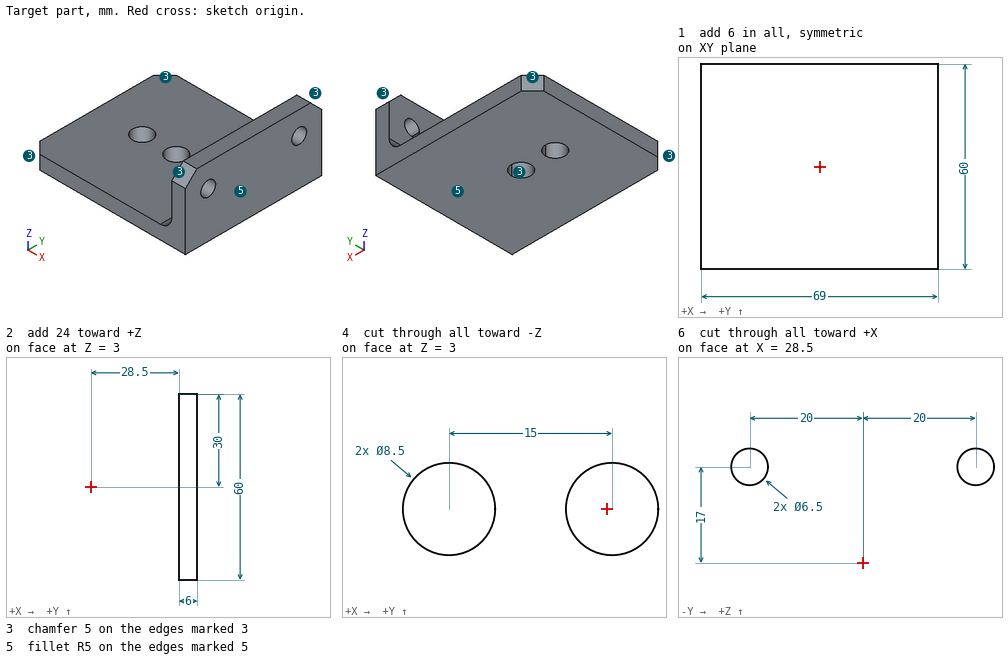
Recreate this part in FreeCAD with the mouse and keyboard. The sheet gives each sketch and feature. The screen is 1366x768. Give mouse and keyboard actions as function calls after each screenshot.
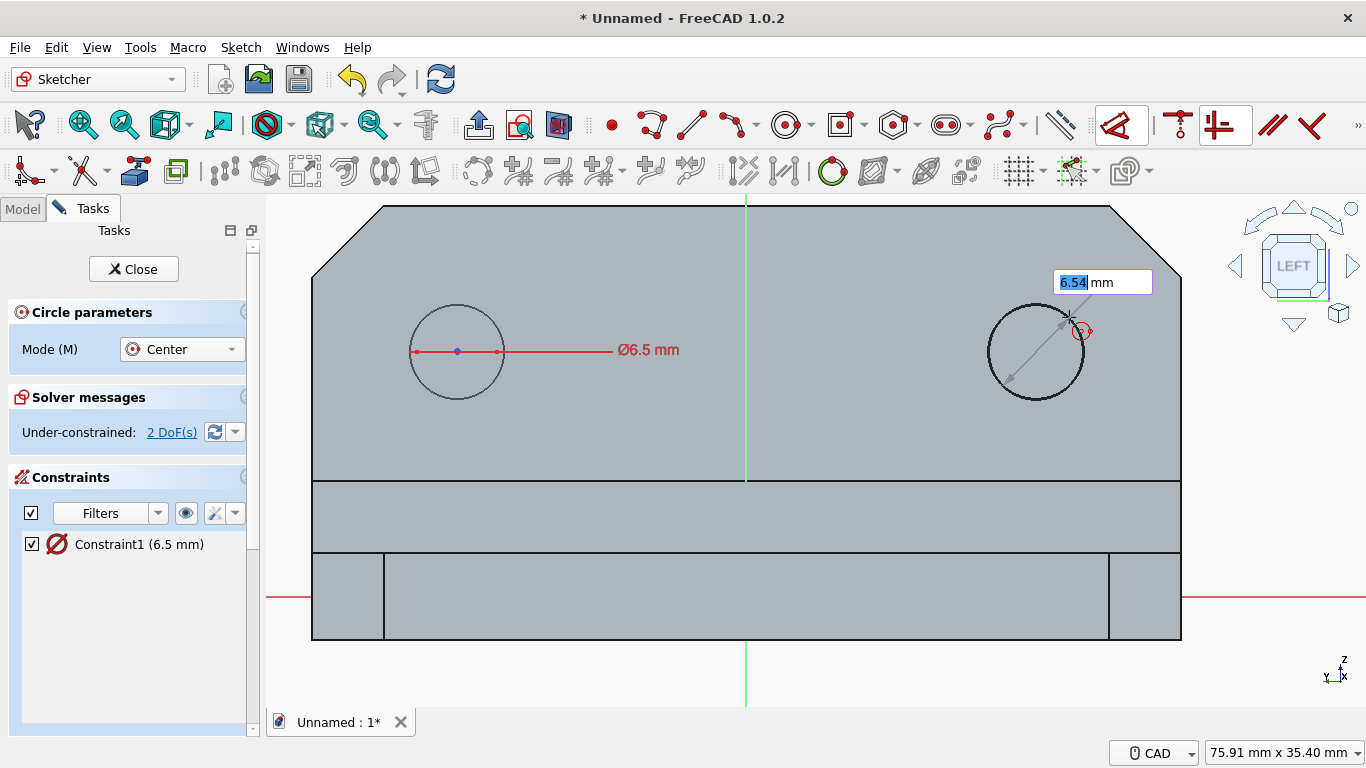
text(6.5)
key(Return)
key(Escape)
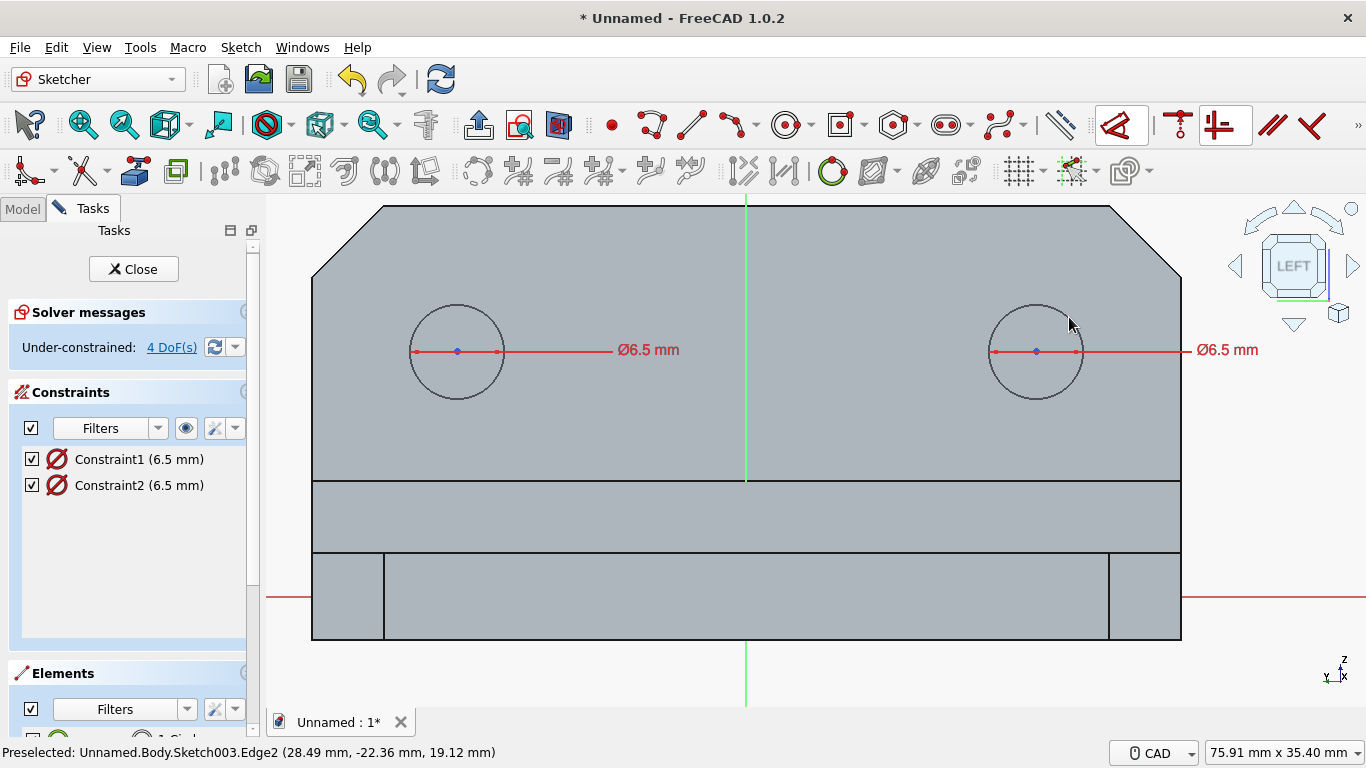
click(457, 352)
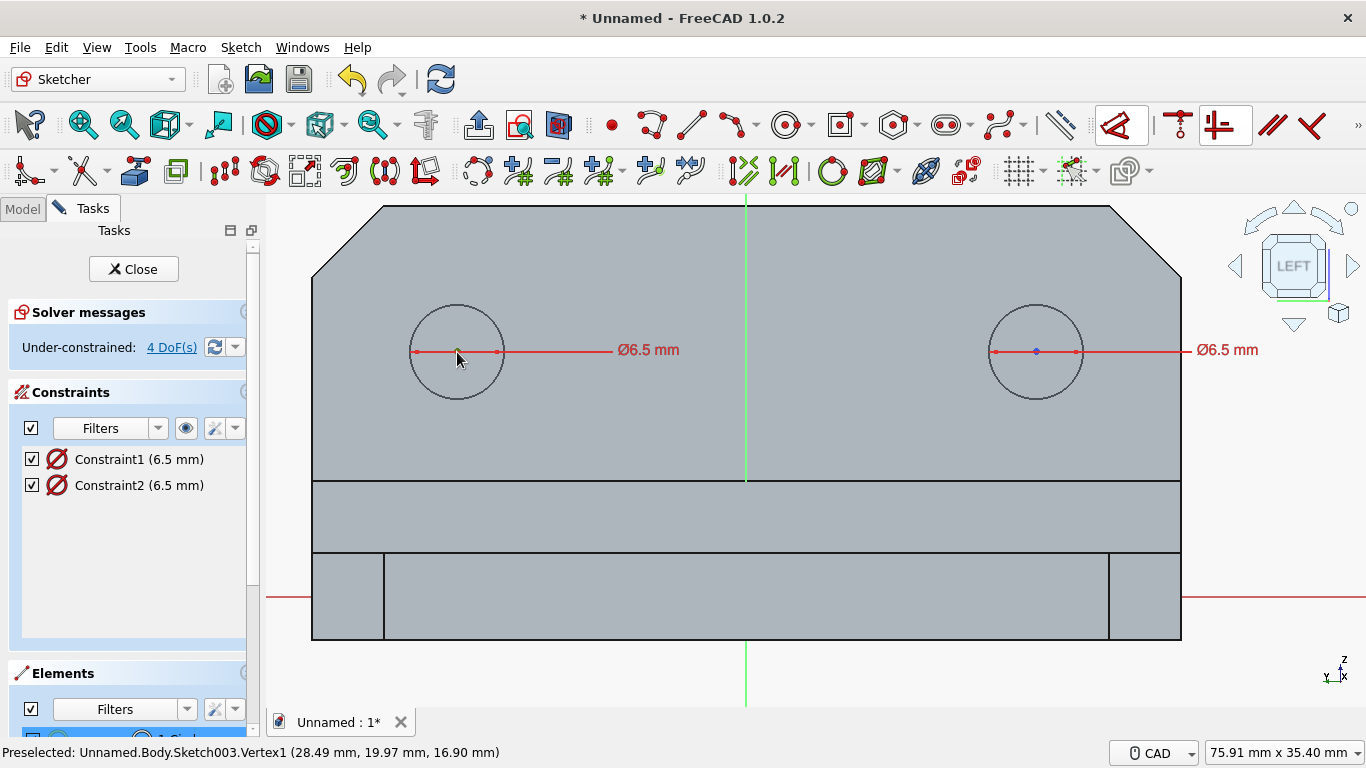
click(1036, 352)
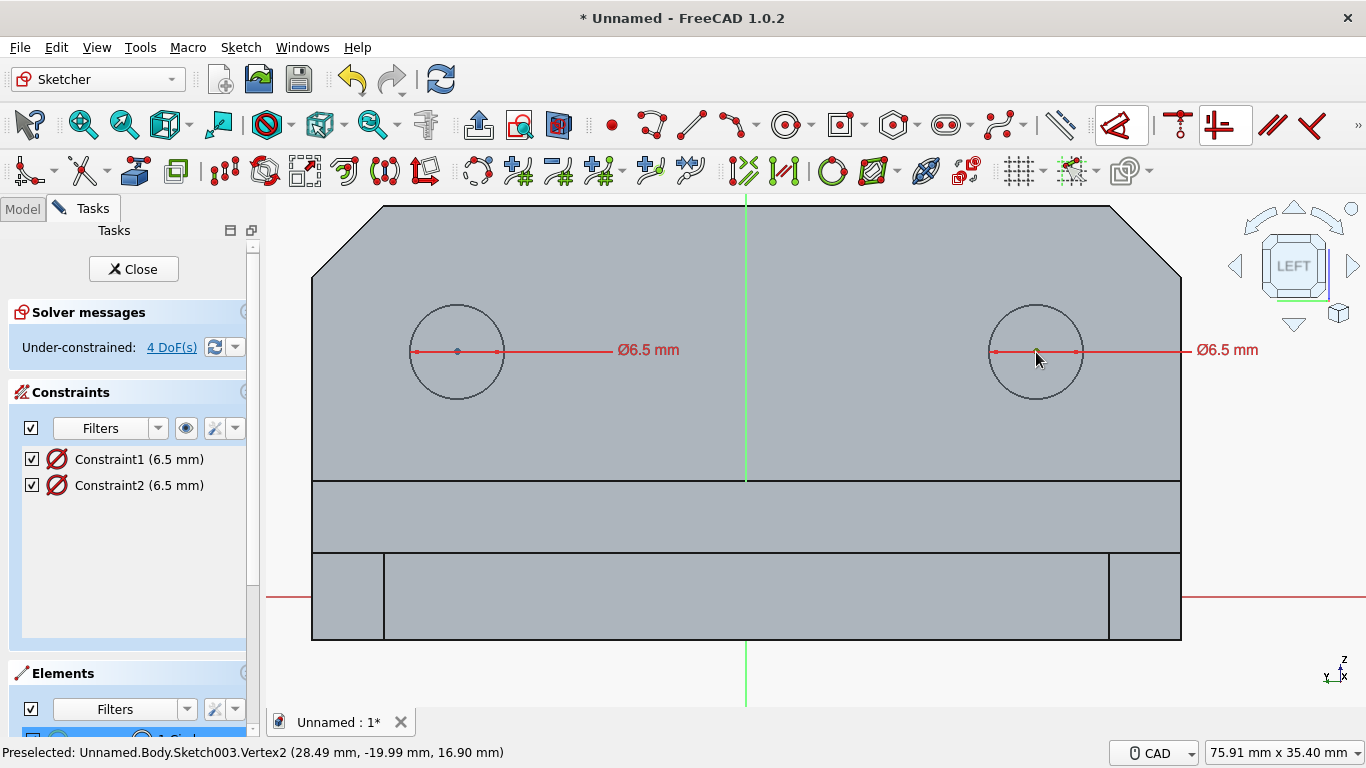
key(h)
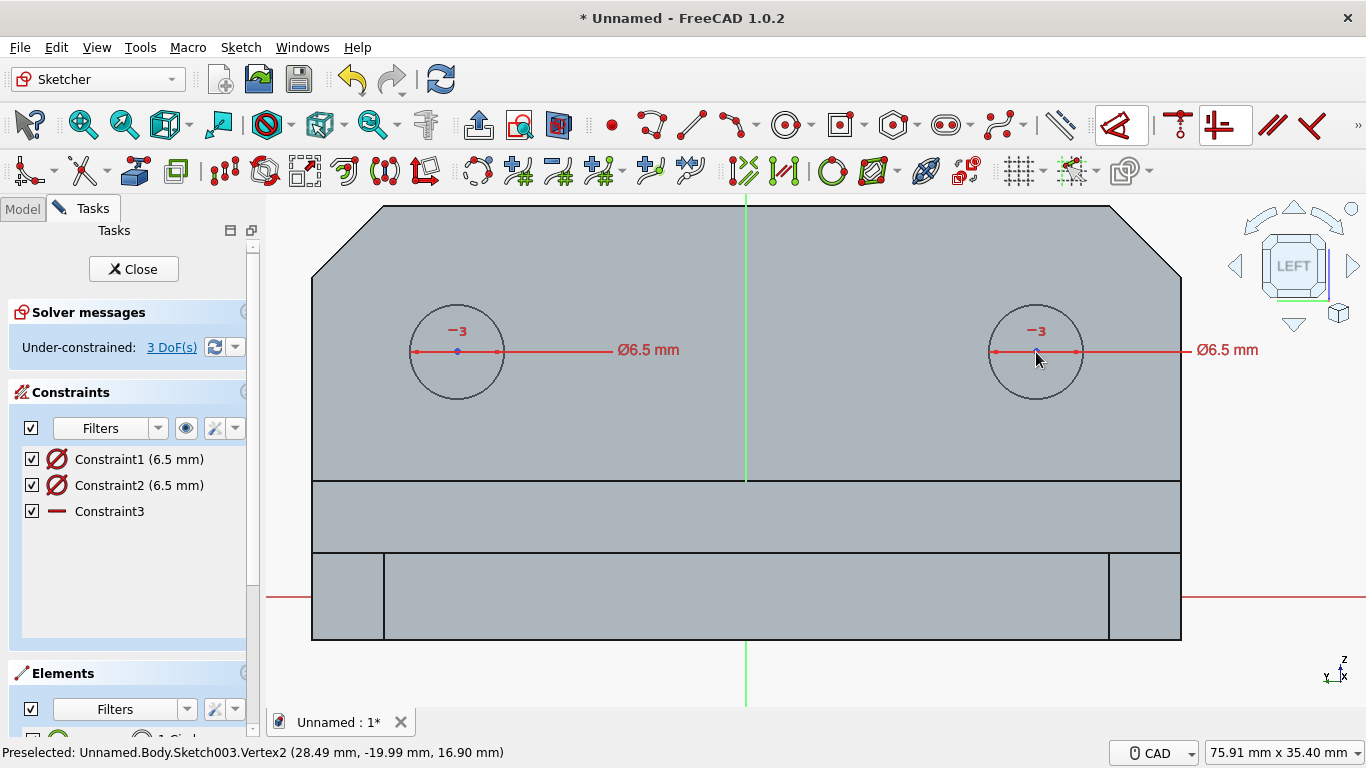
click(457, 352)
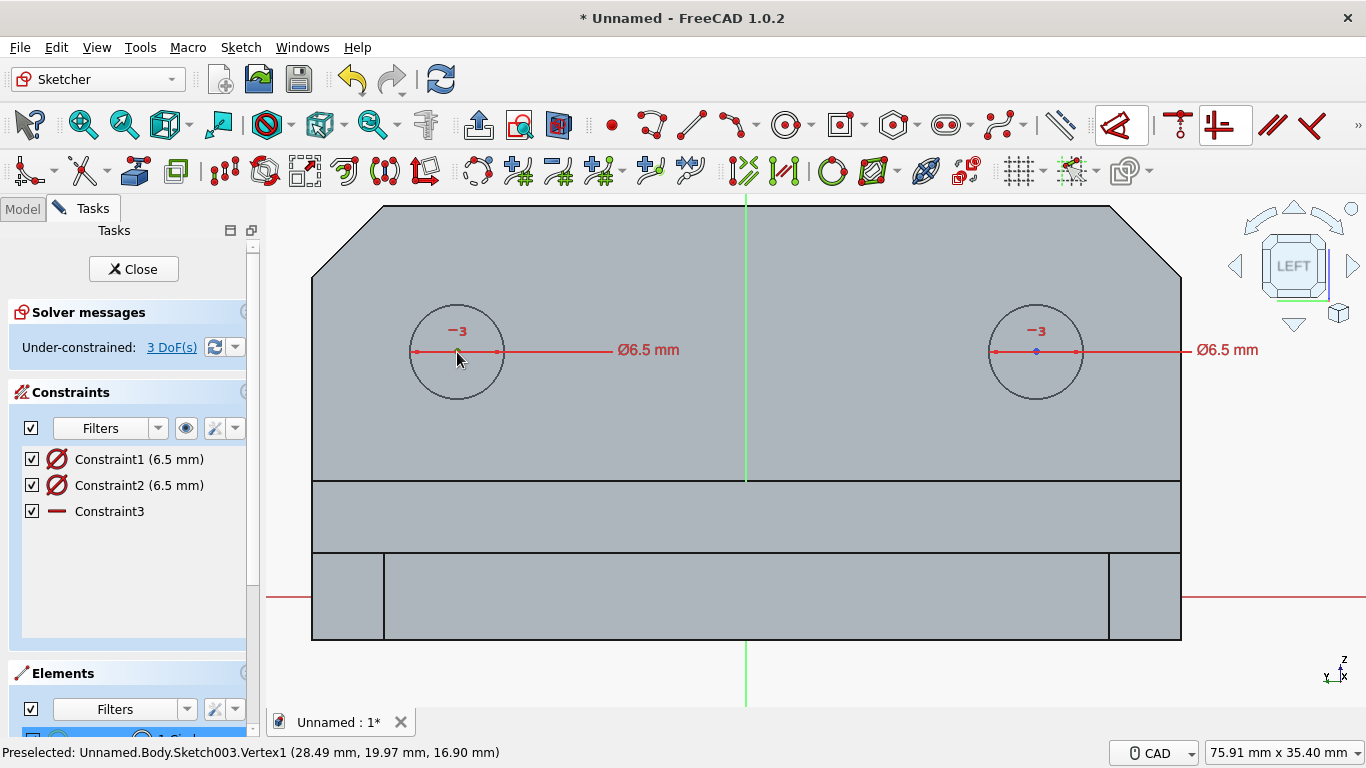
click(1142, 126)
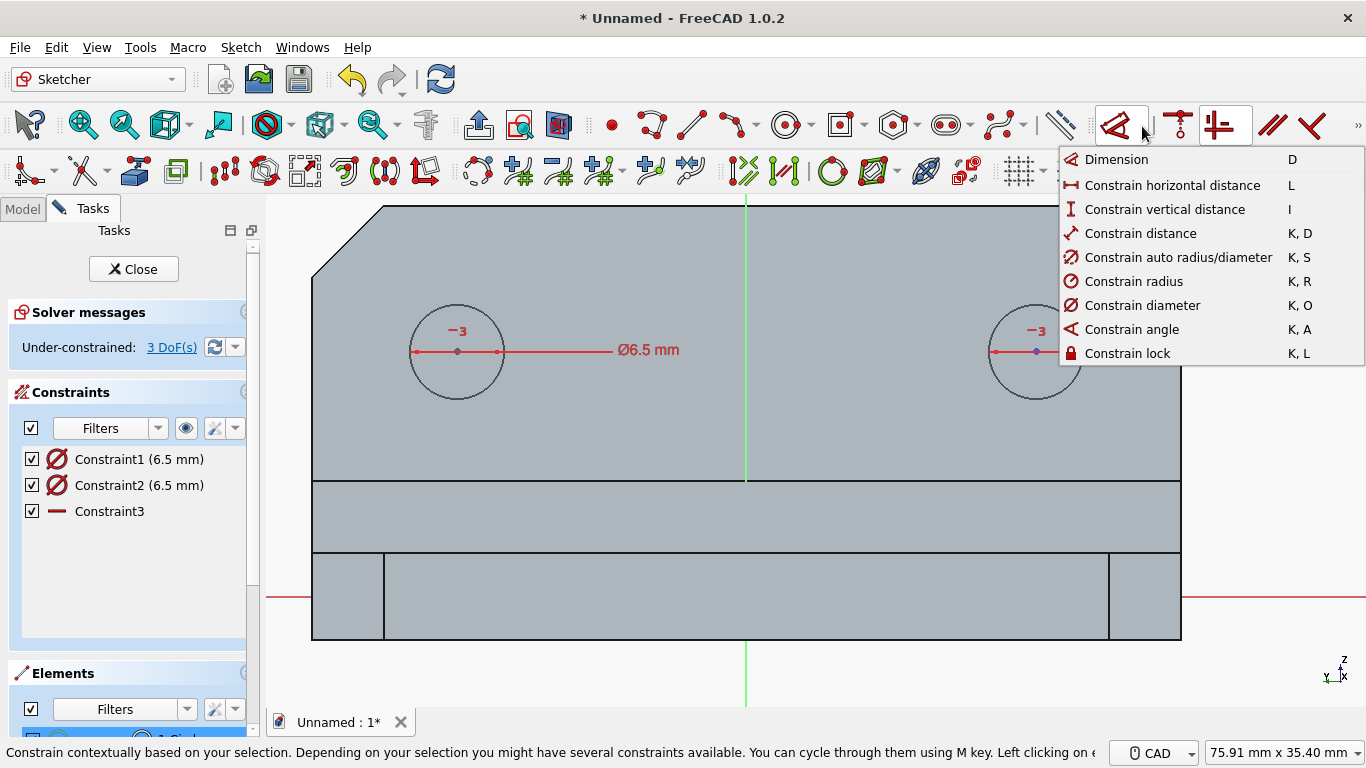
click(1212, 185)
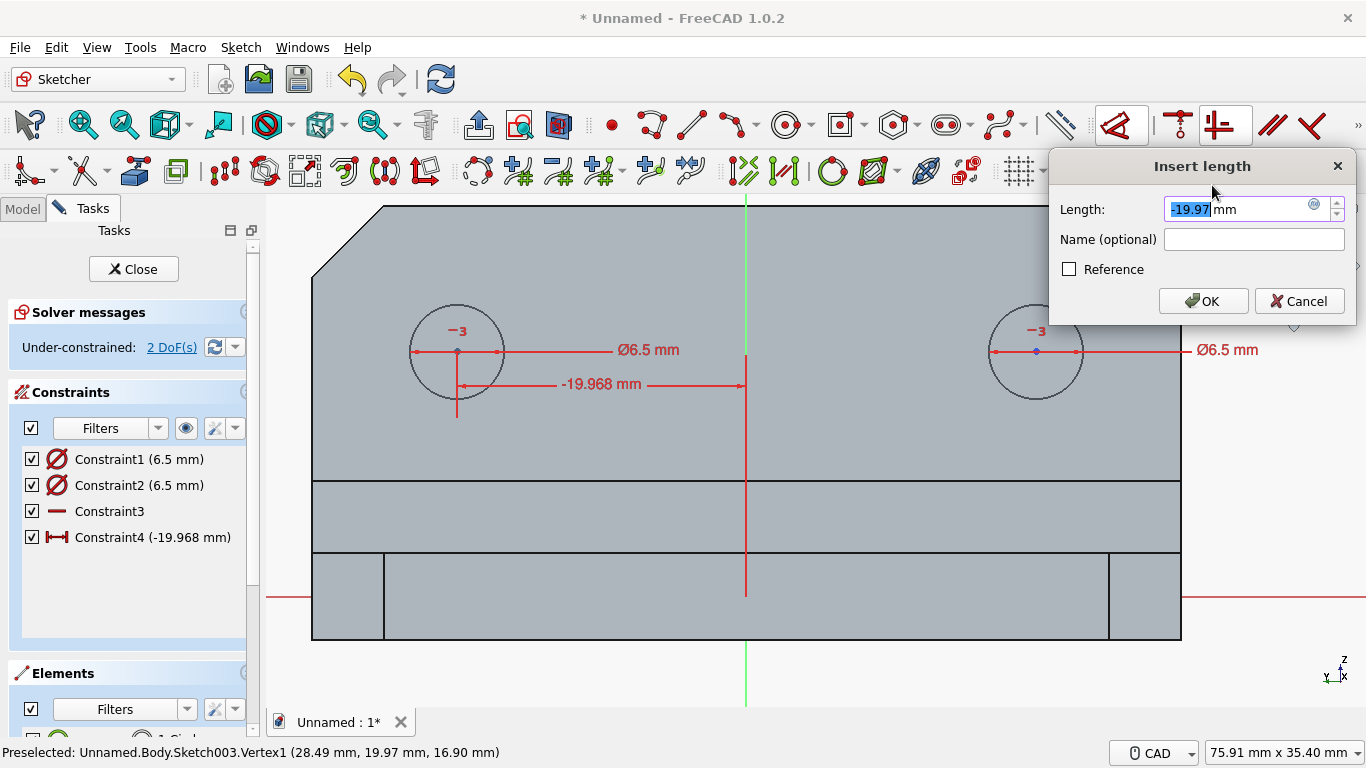
text(-20)
key(Return)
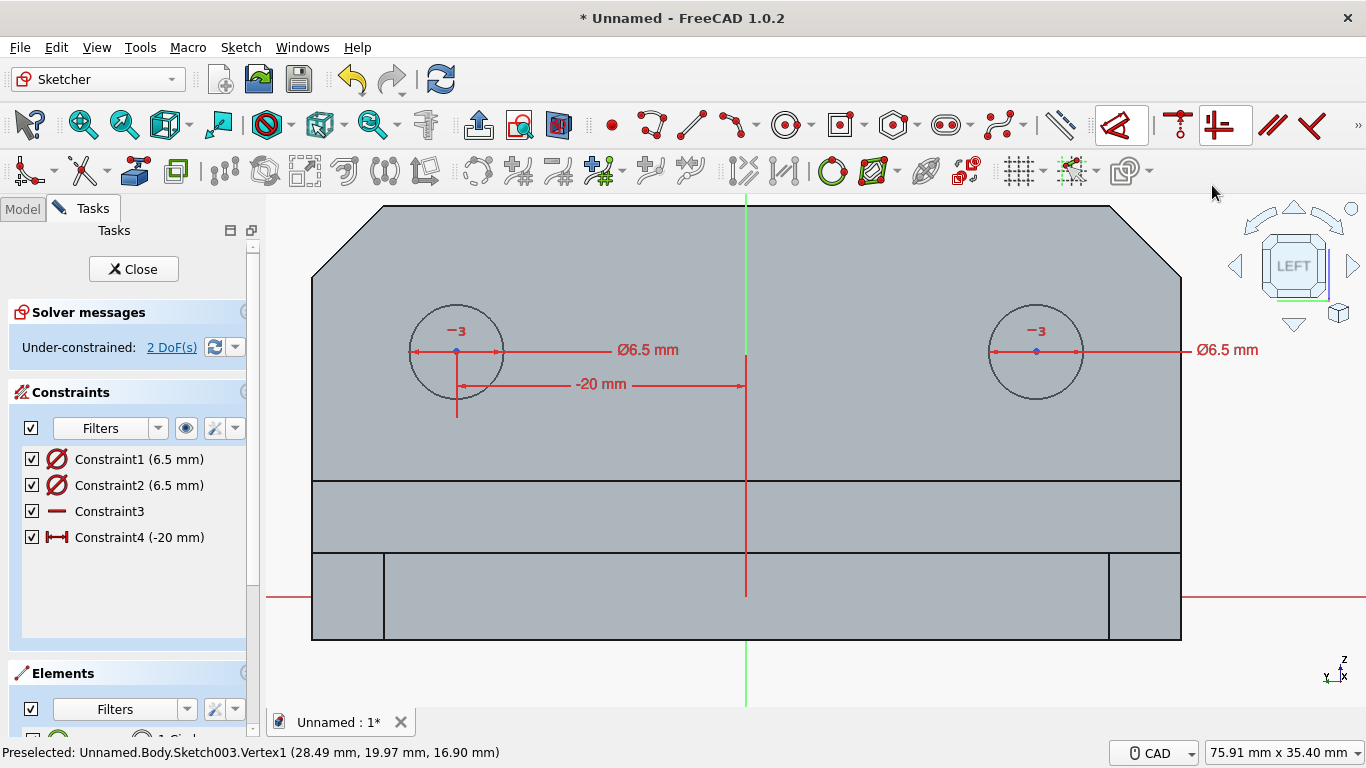
click(457, 352)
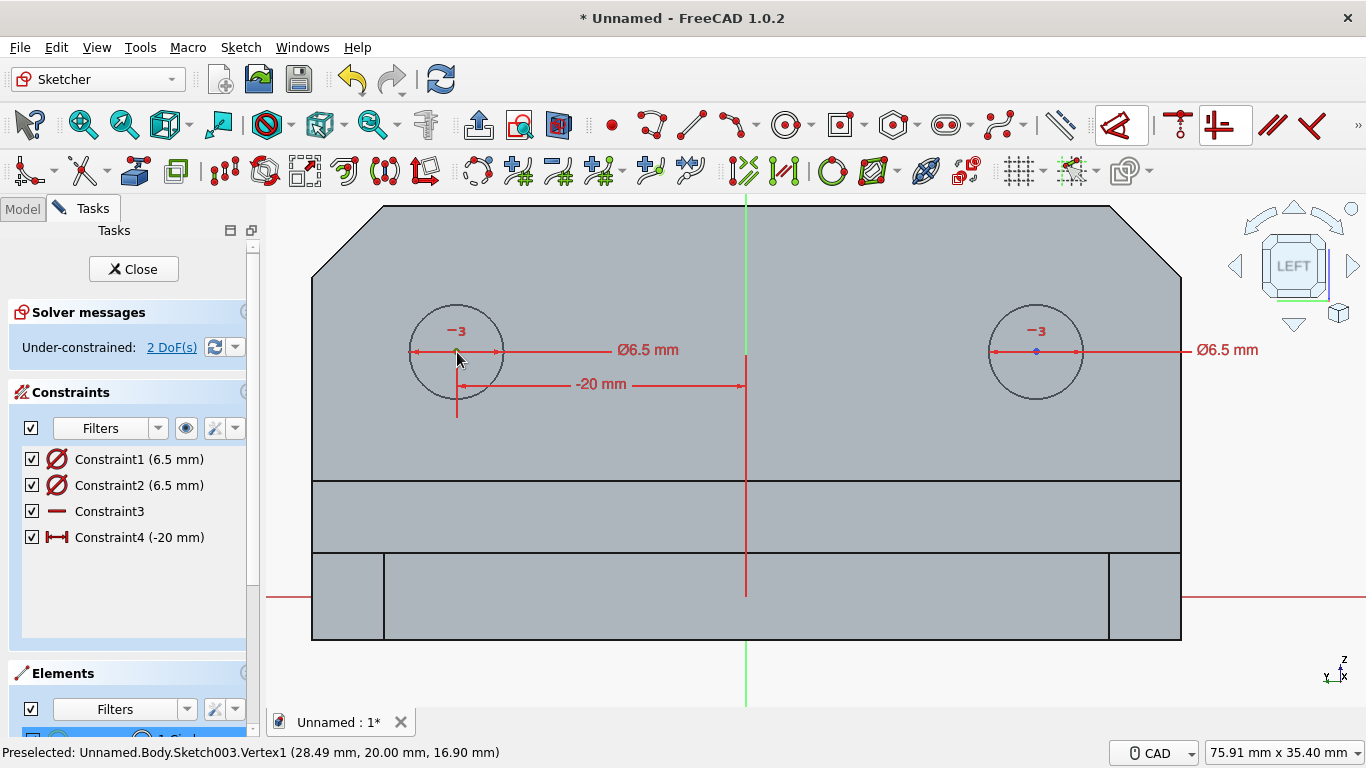
click(1142, 126)